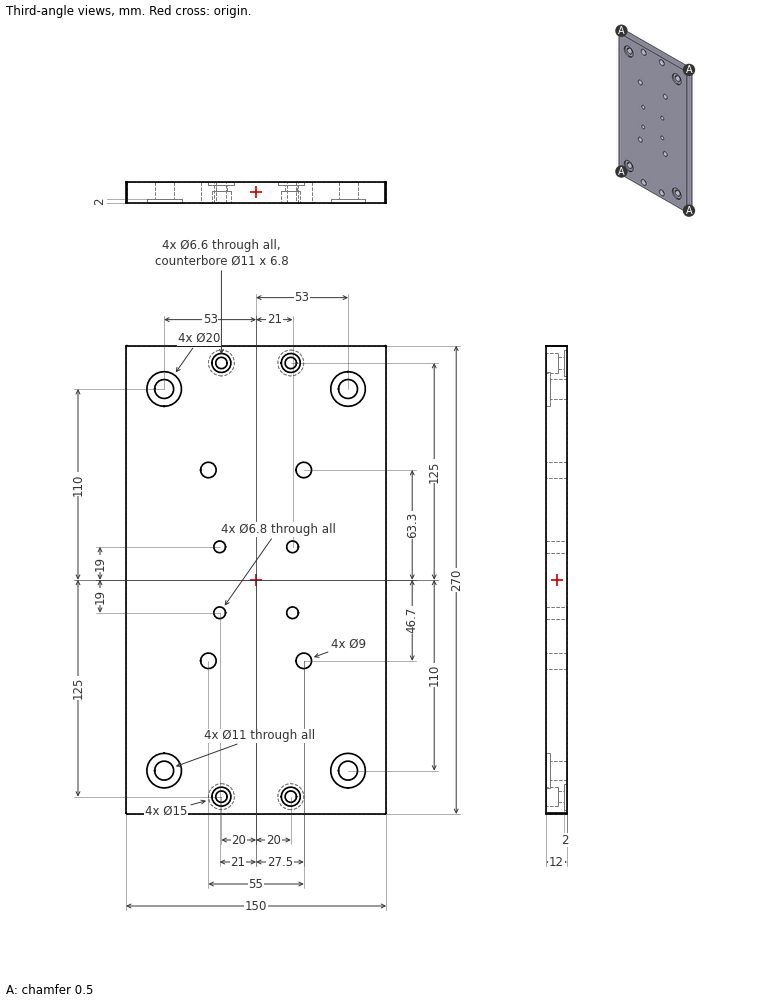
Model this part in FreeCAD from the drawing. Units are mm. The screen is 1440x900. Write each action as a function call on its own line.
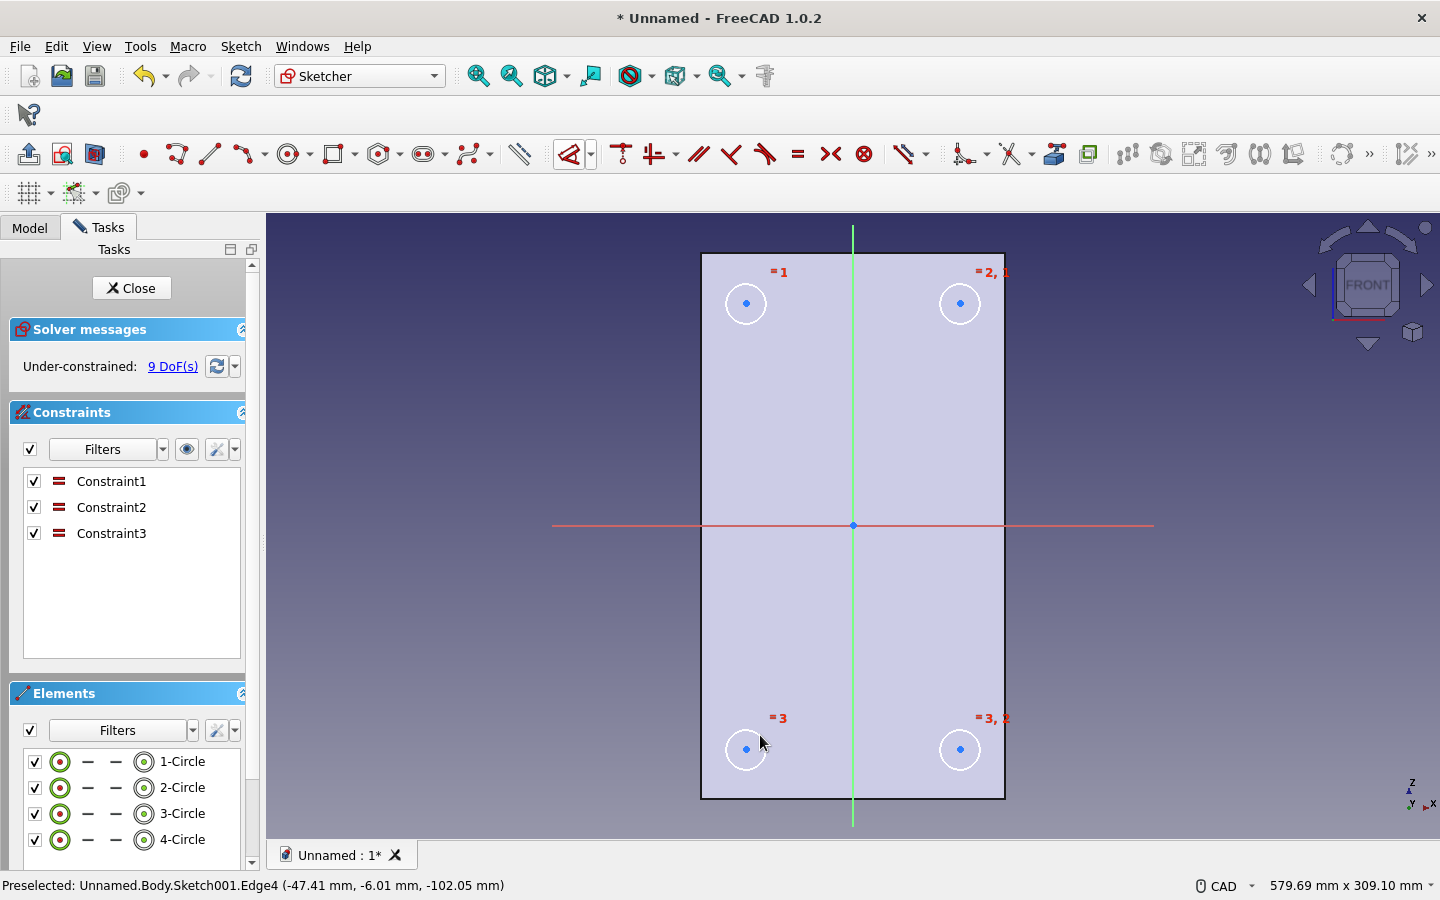
click(746, 304)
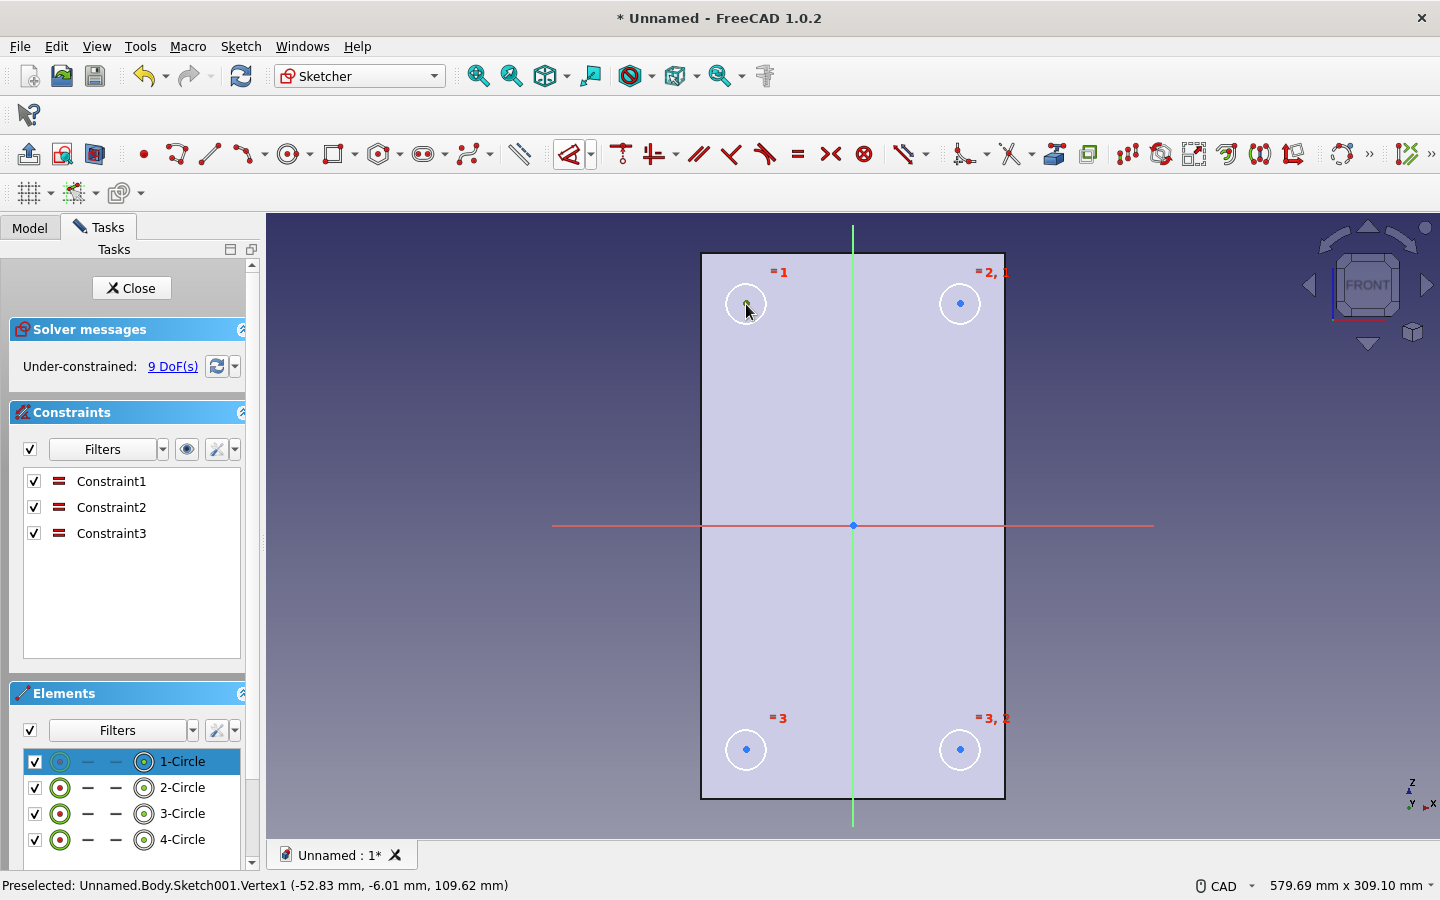
click(960, 304)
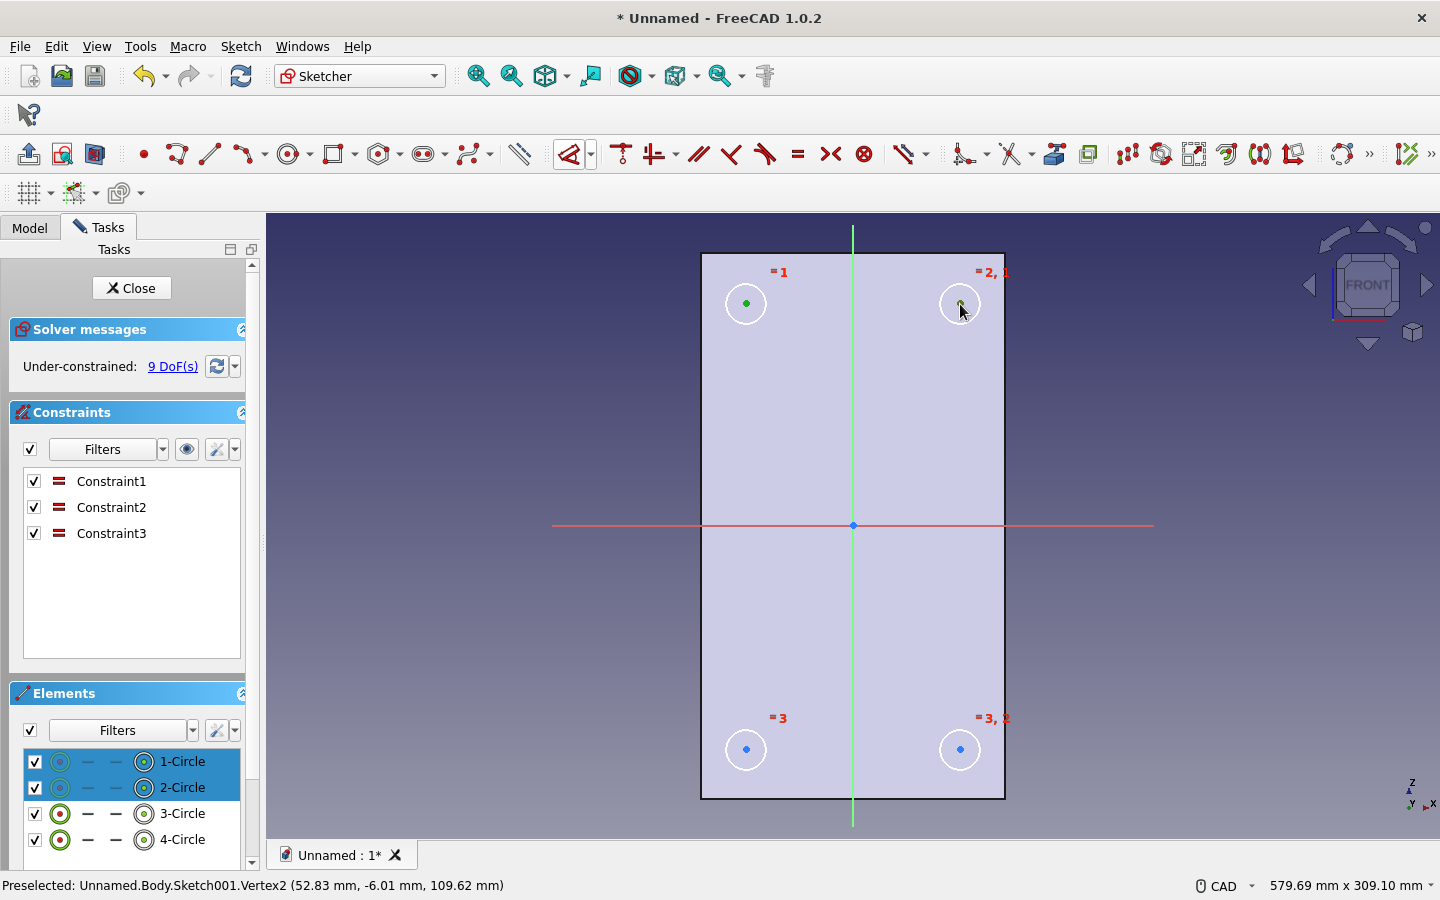
key(h)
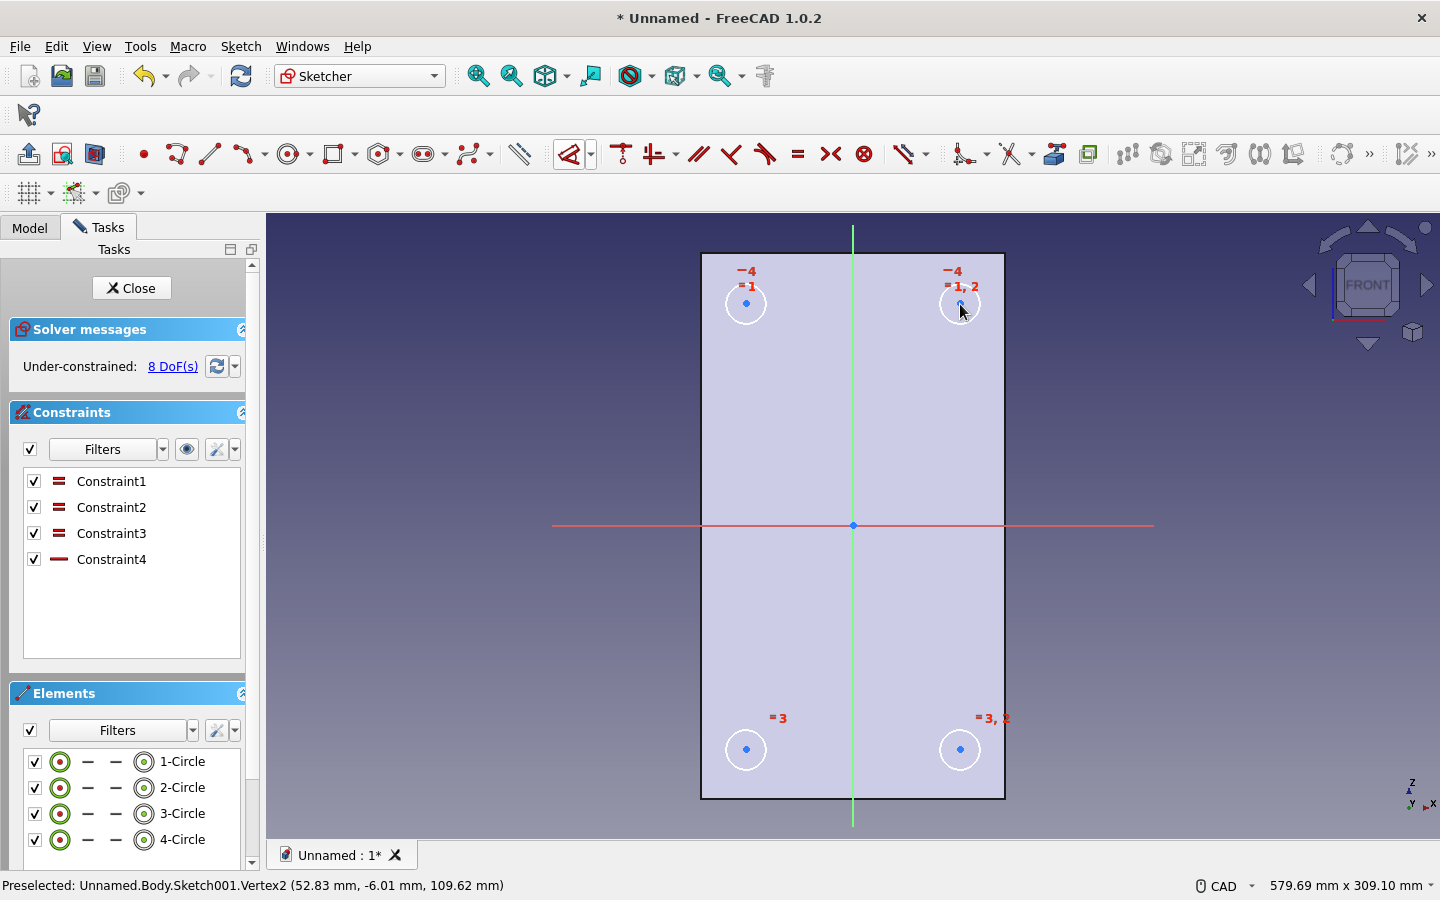
click(960, 304)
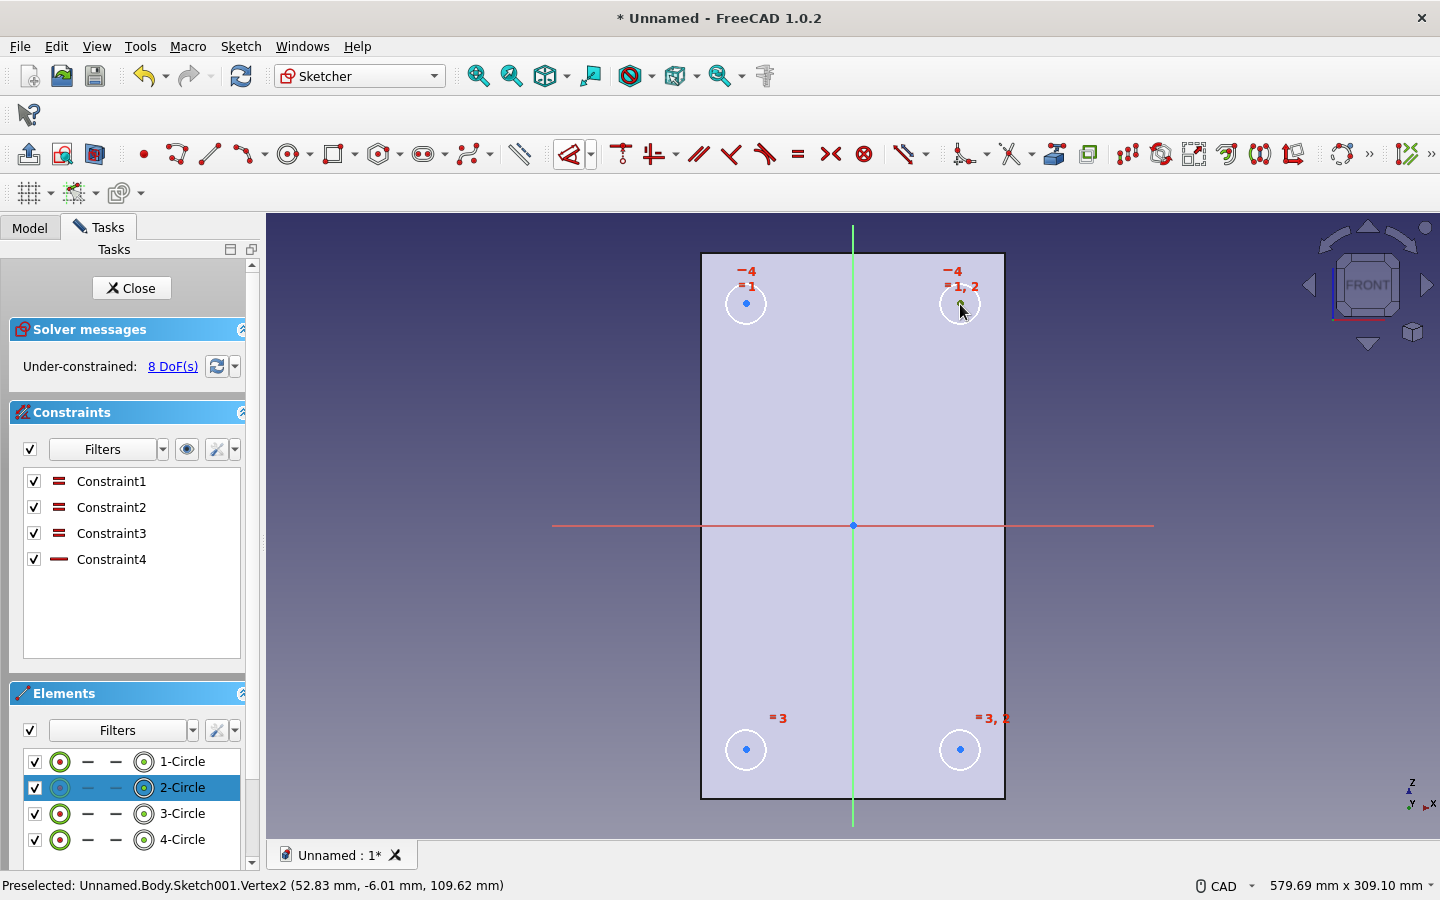
click(960, 750)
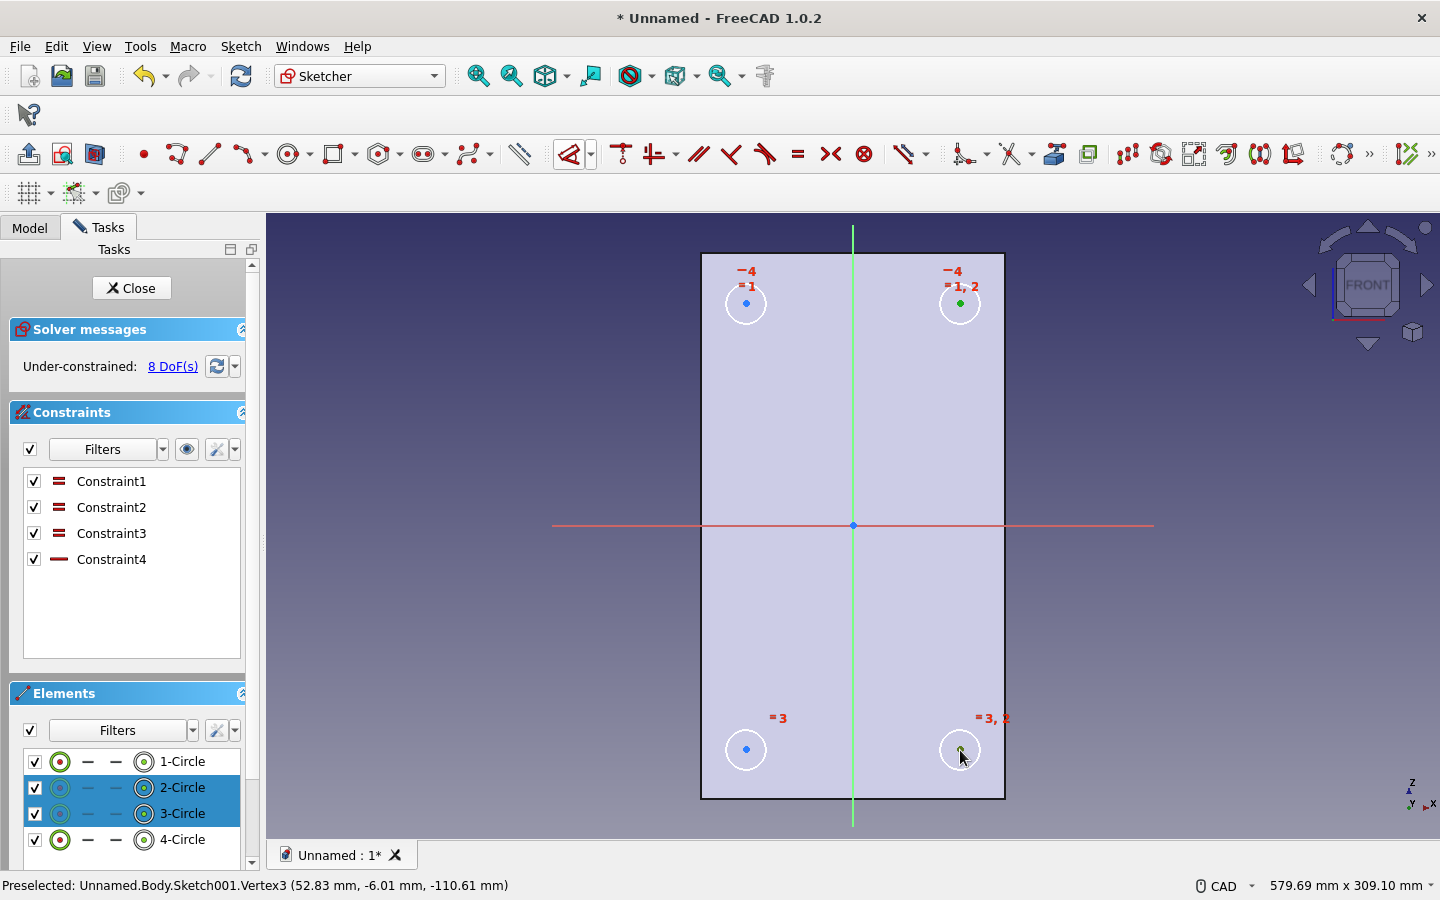
key(v)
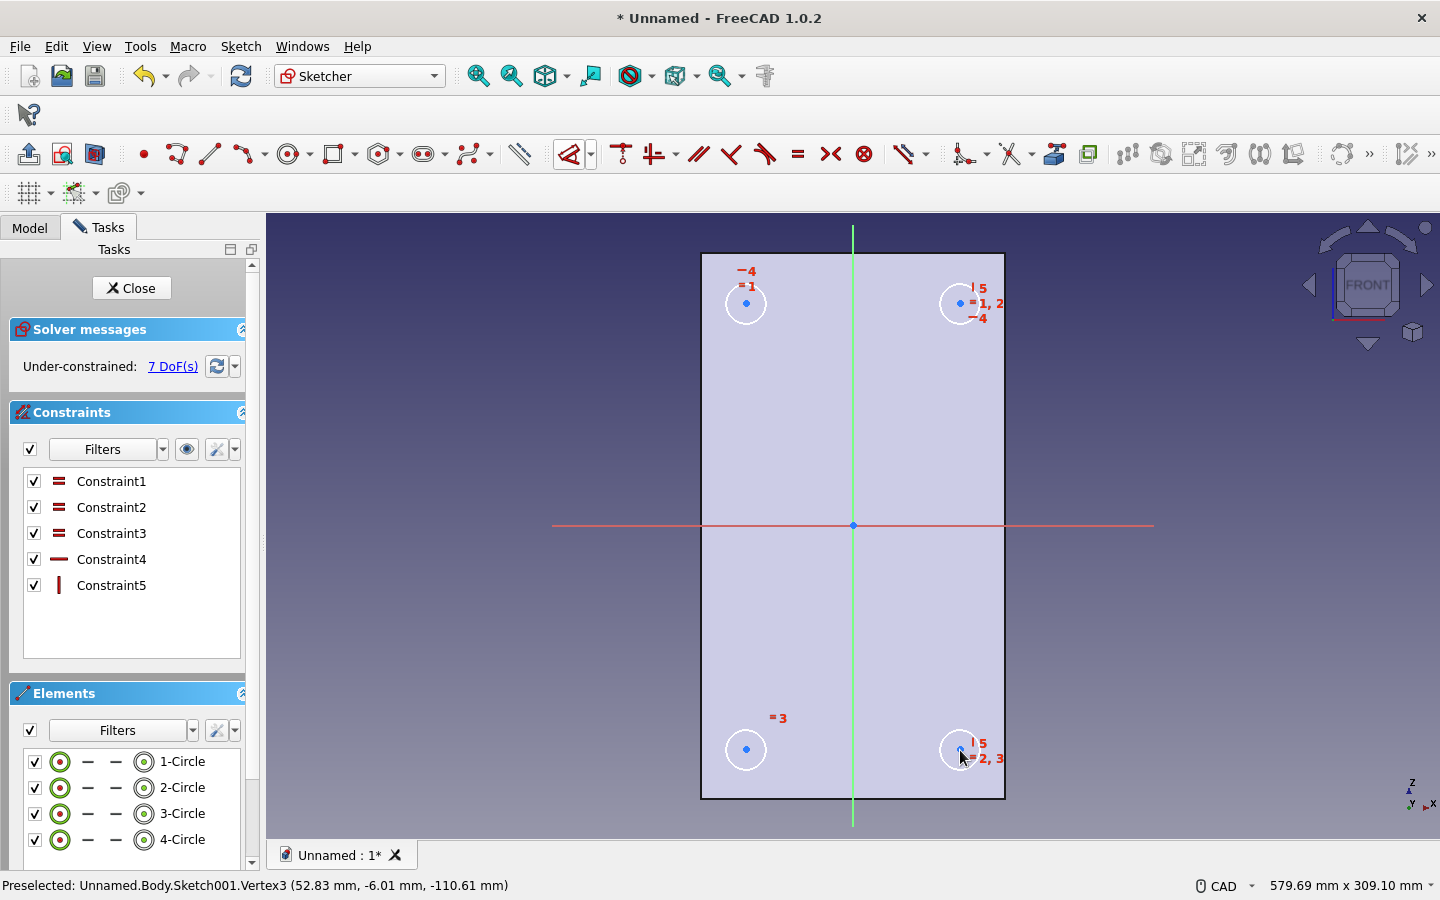
click(746, 304)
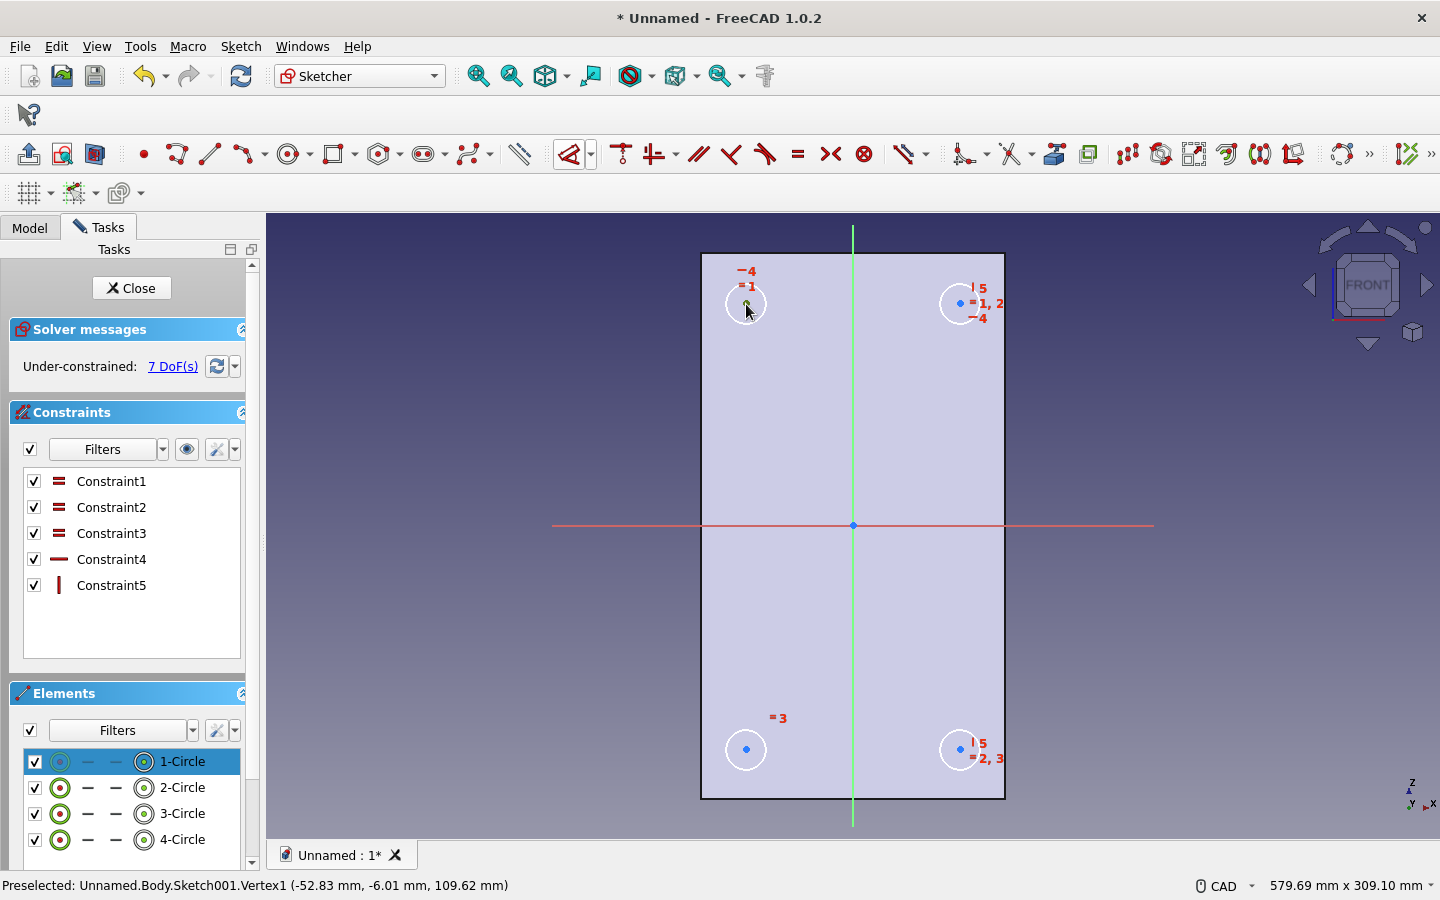
click(746, 750)